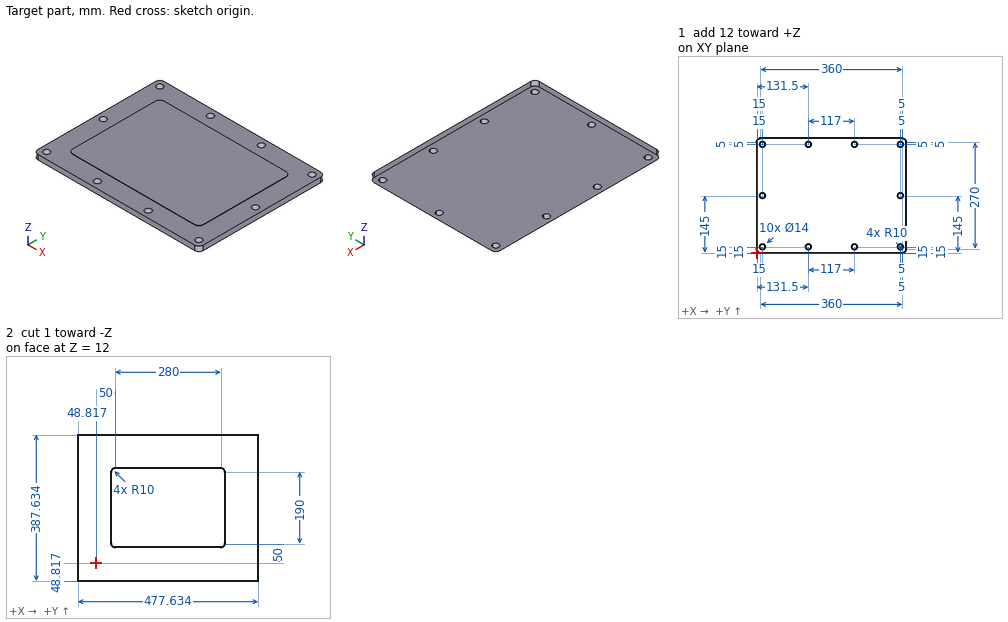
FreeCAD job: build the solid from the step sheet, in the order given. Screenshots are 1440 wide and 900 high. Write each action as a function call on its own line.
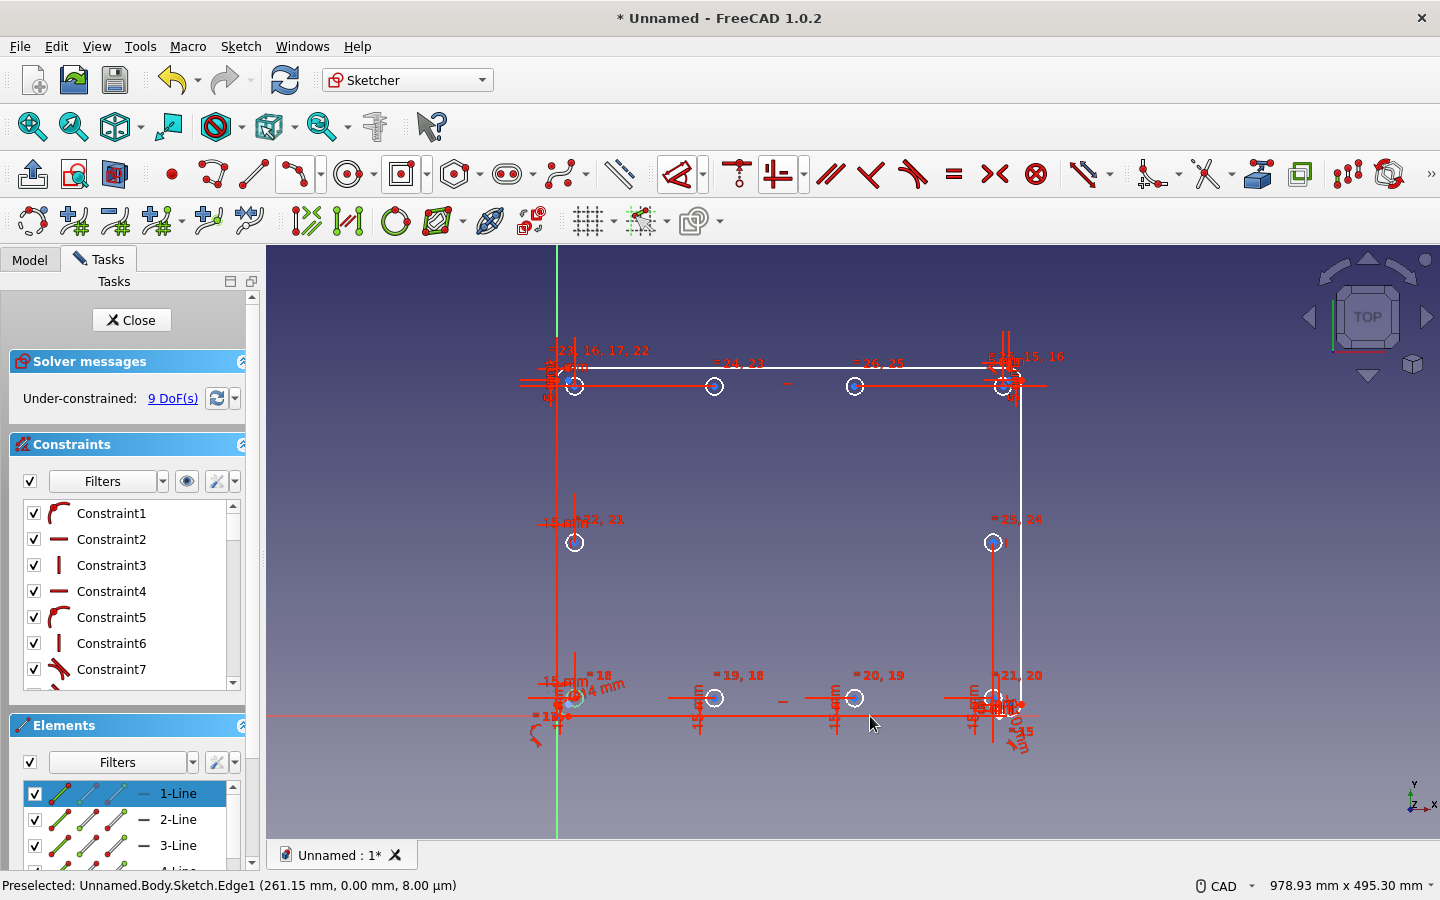
click(702, 174)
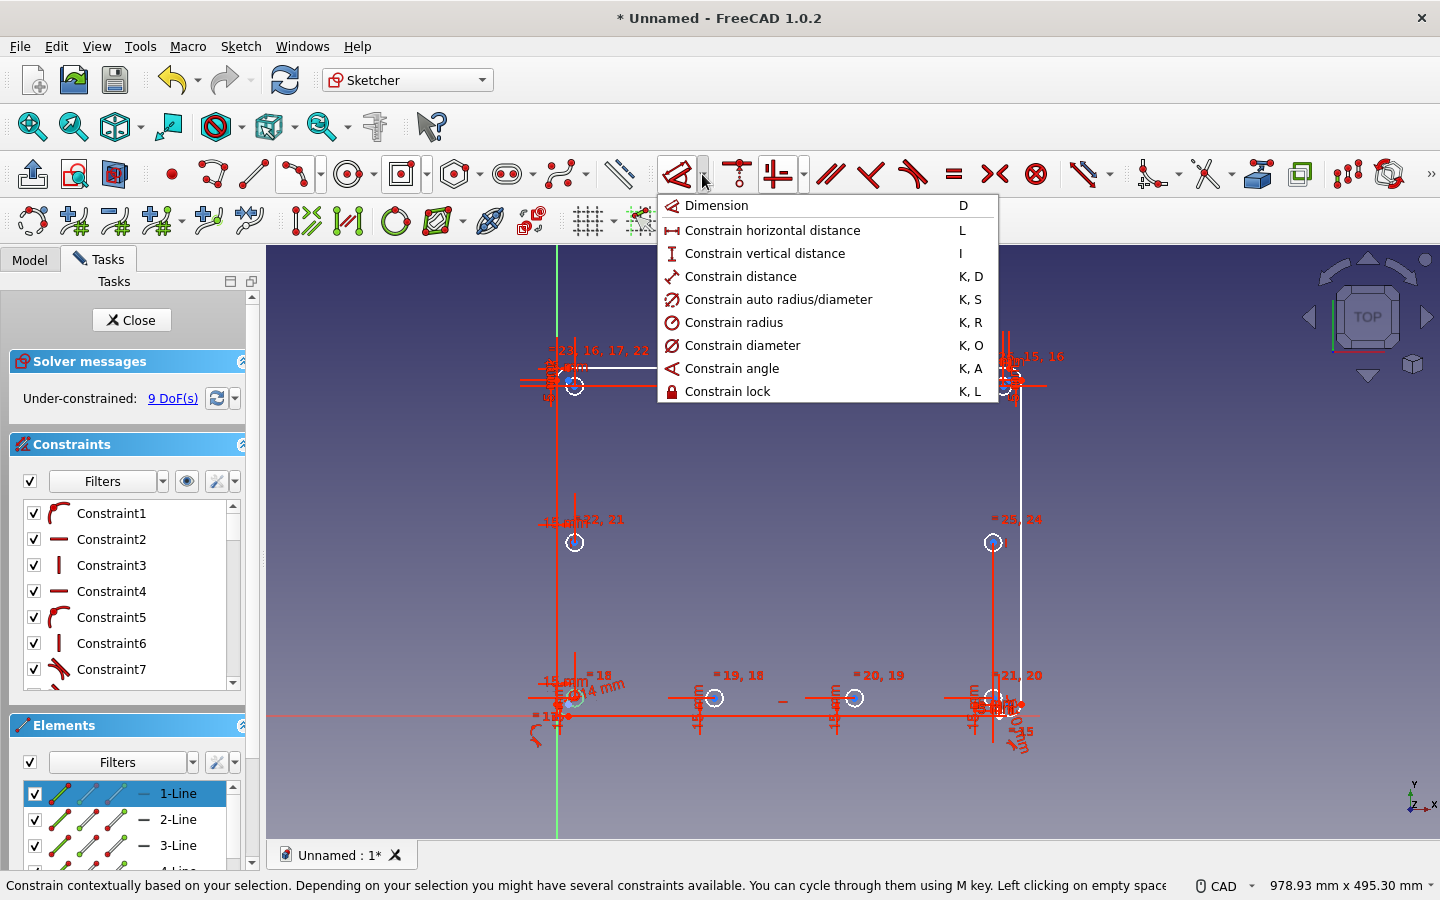
click(828, 230)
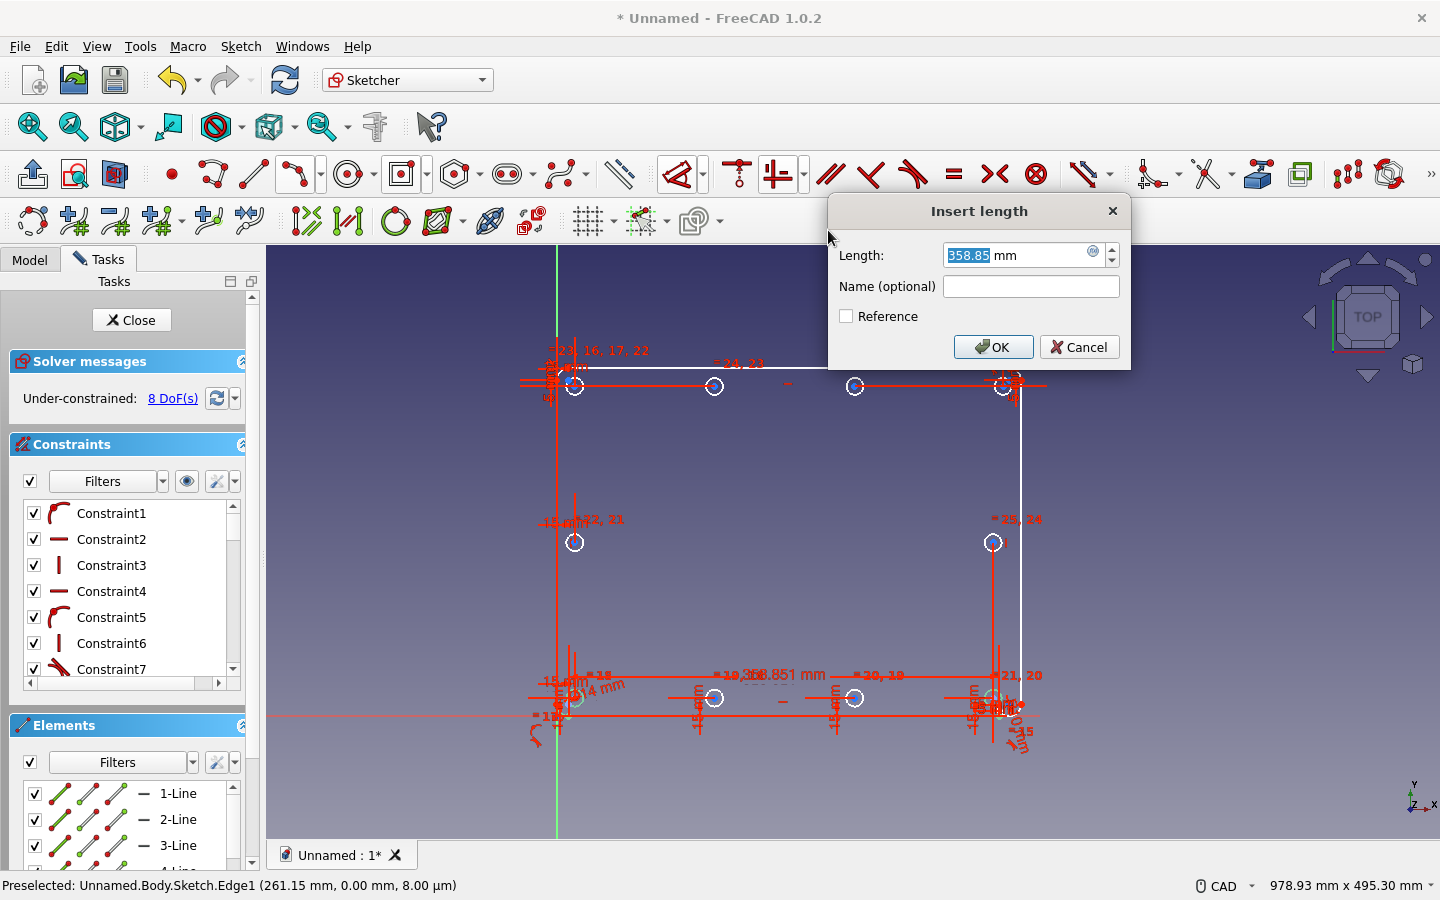
text(360)
key(Return)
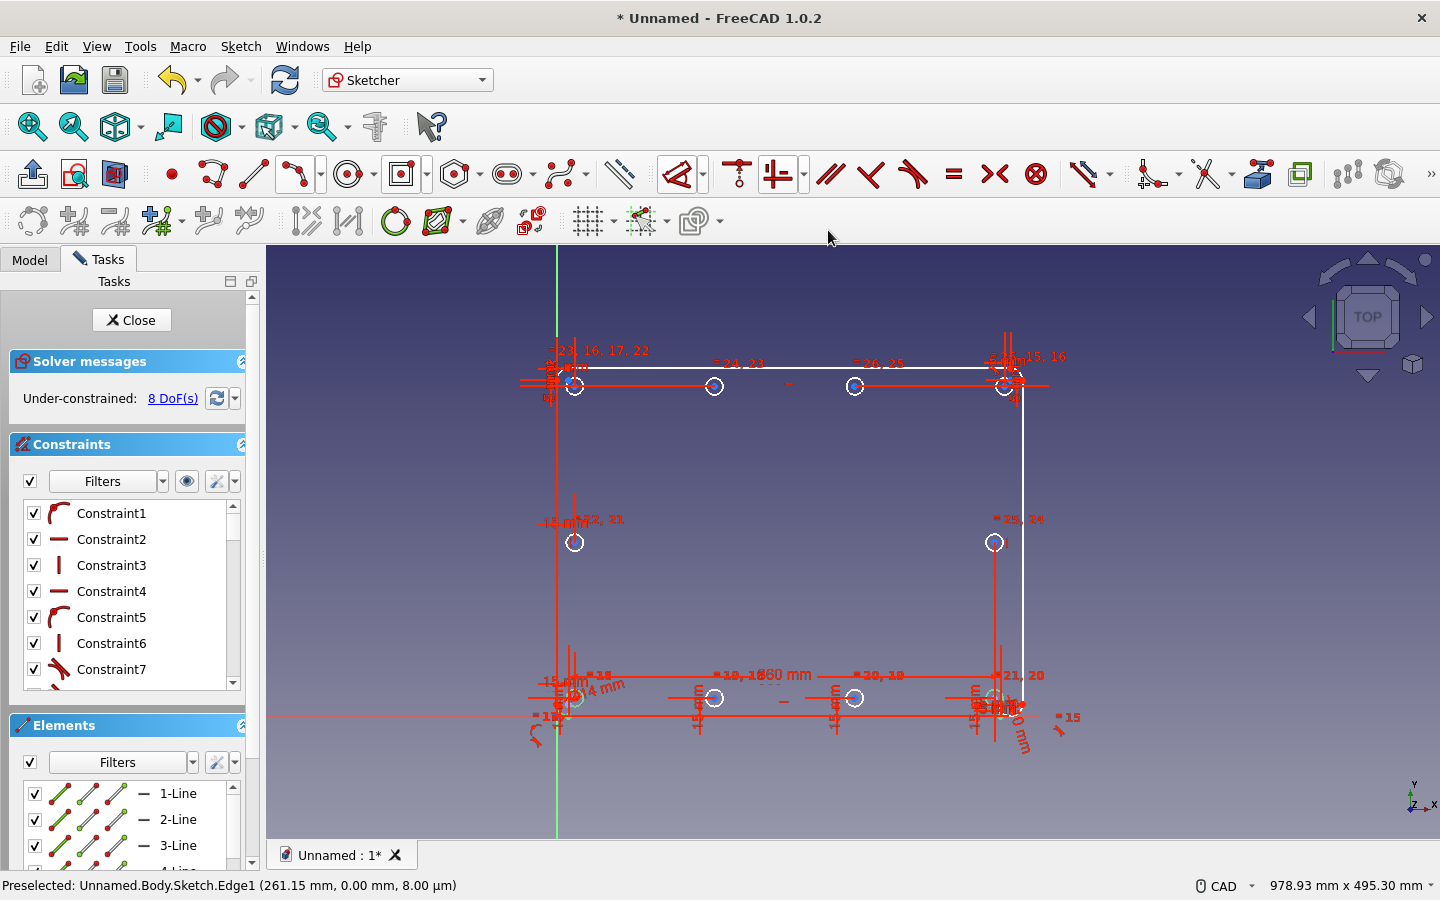
click(1023, 607)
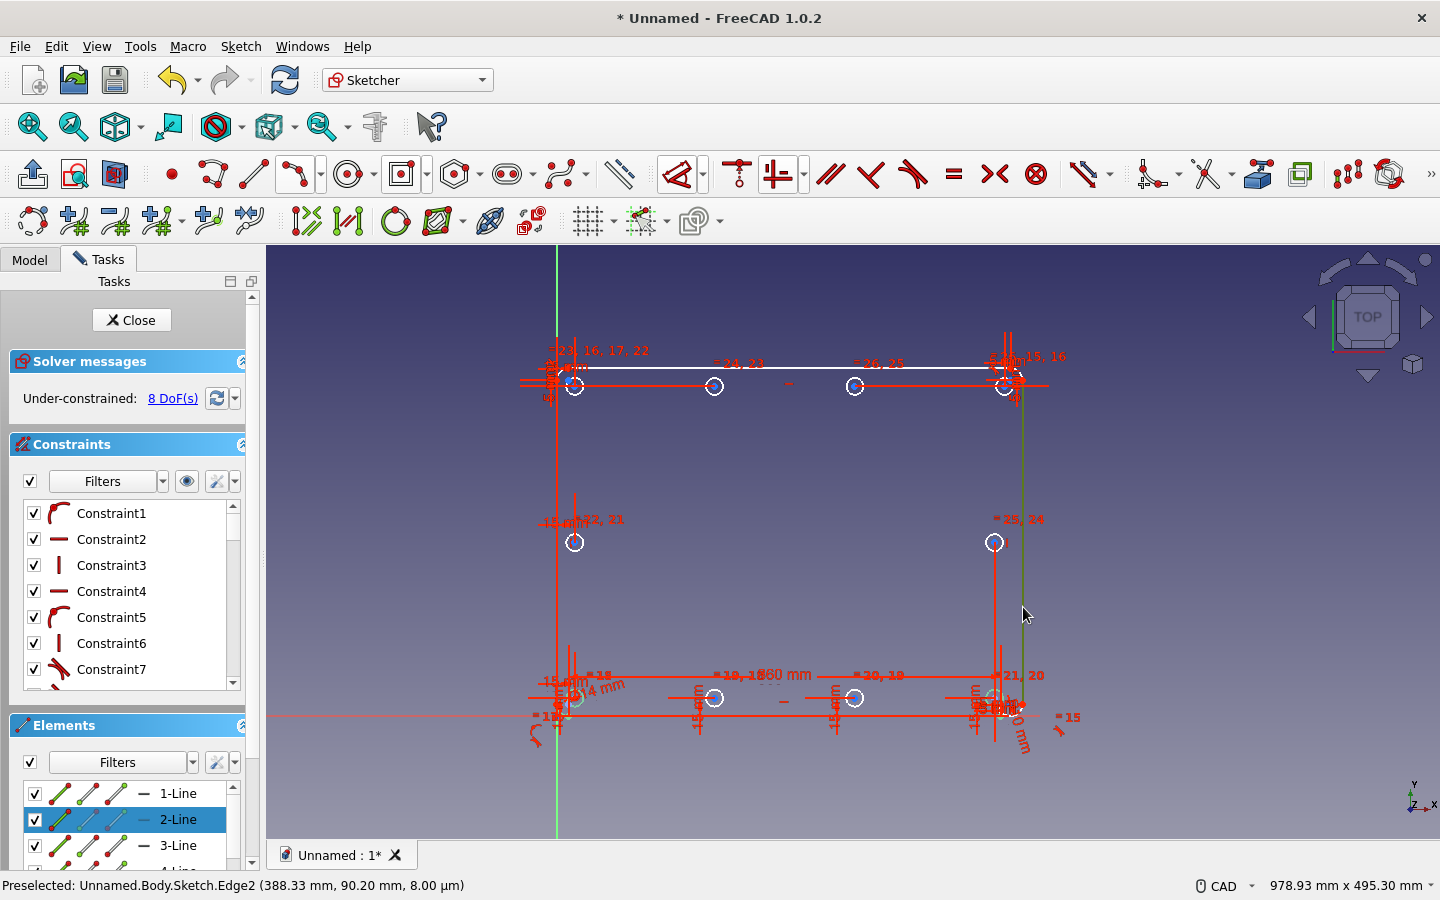
key(i)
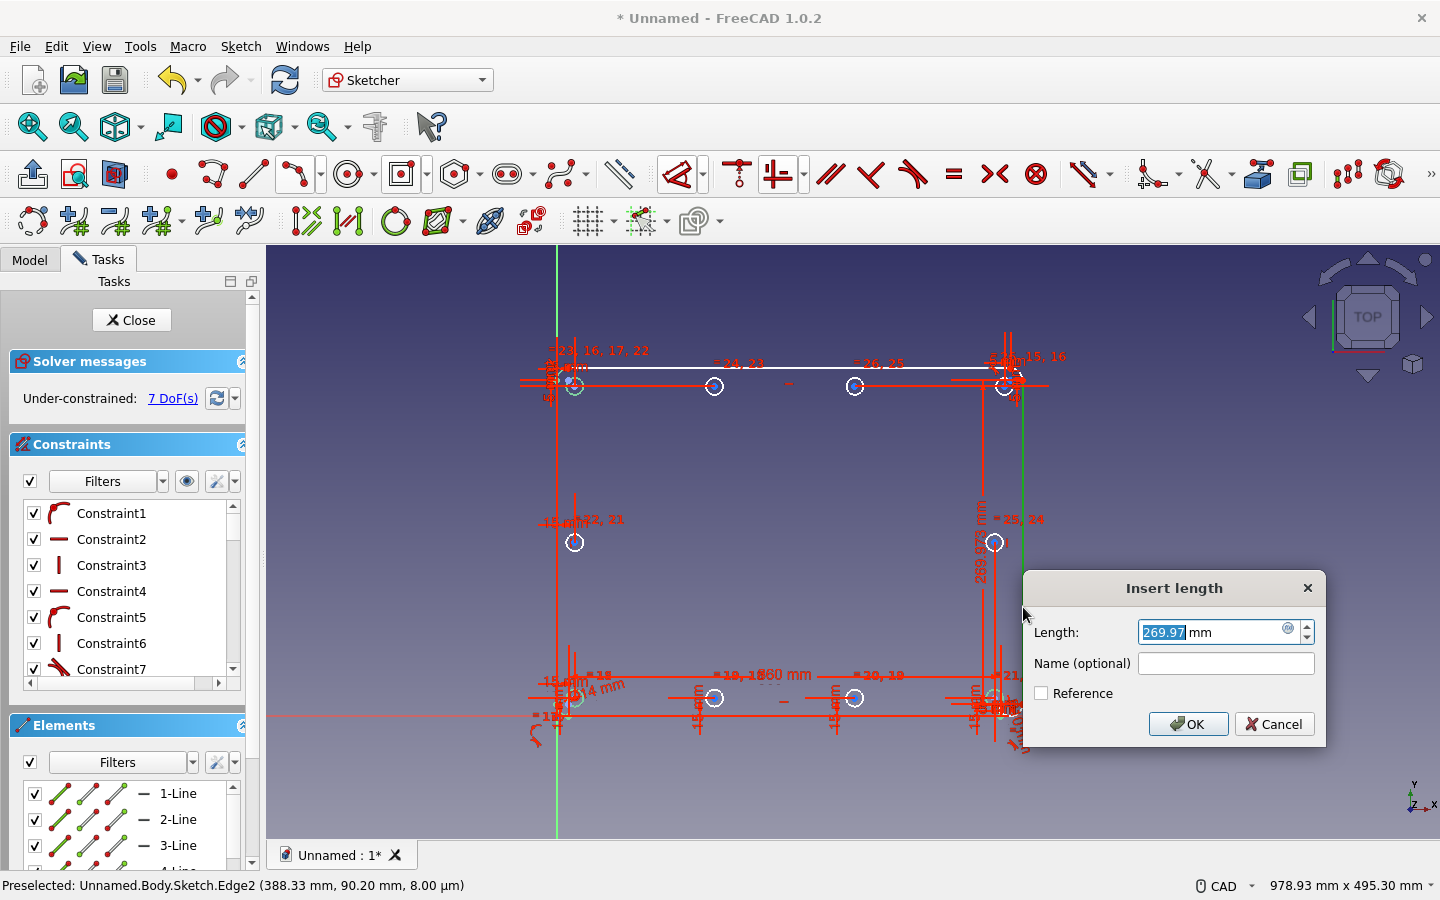
text(270)
key(Return)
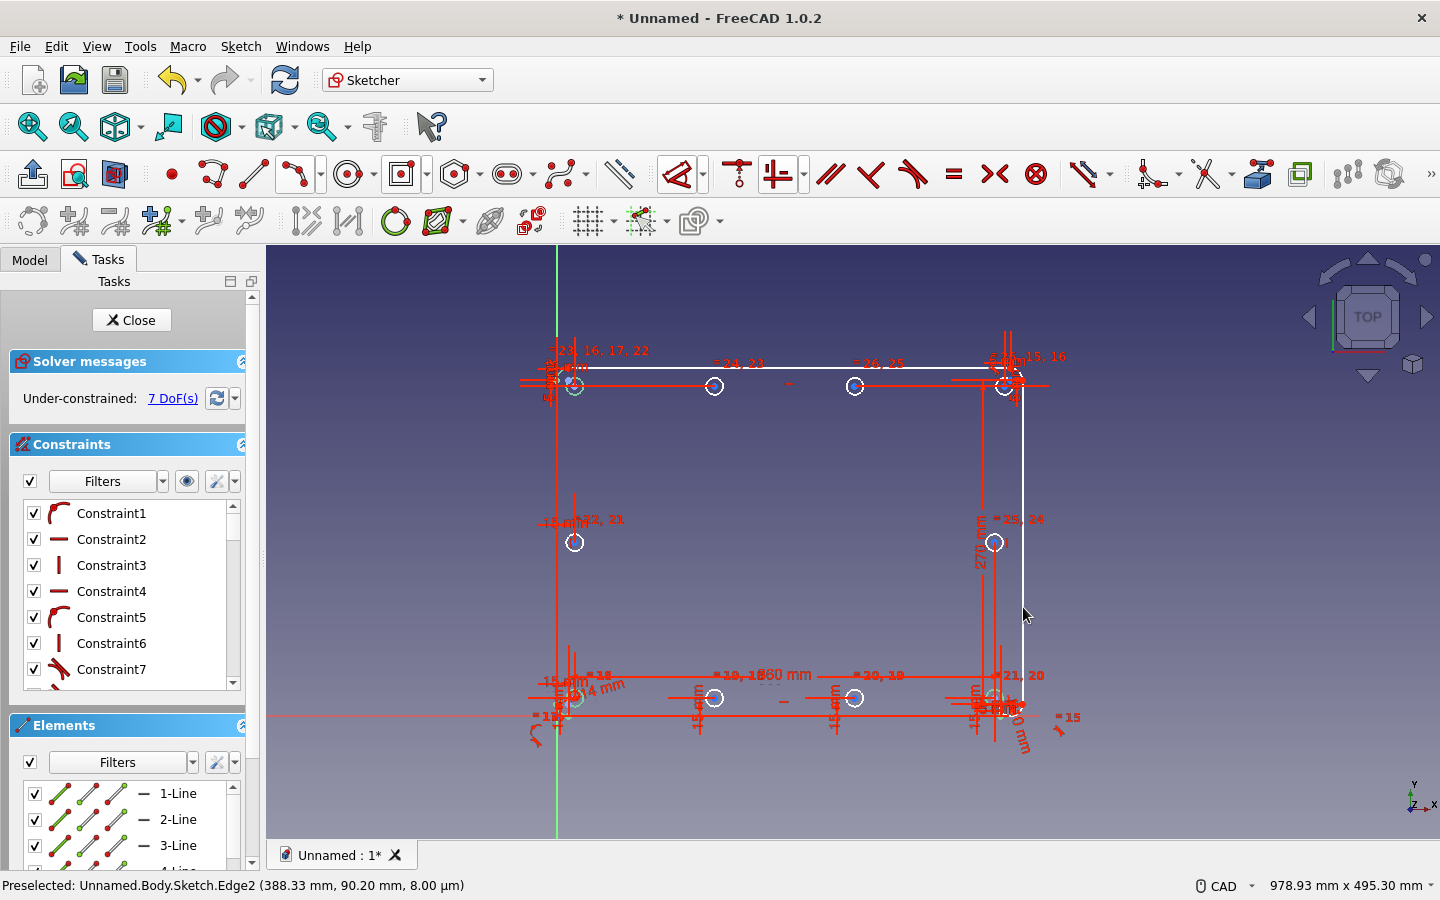
click(701, 368)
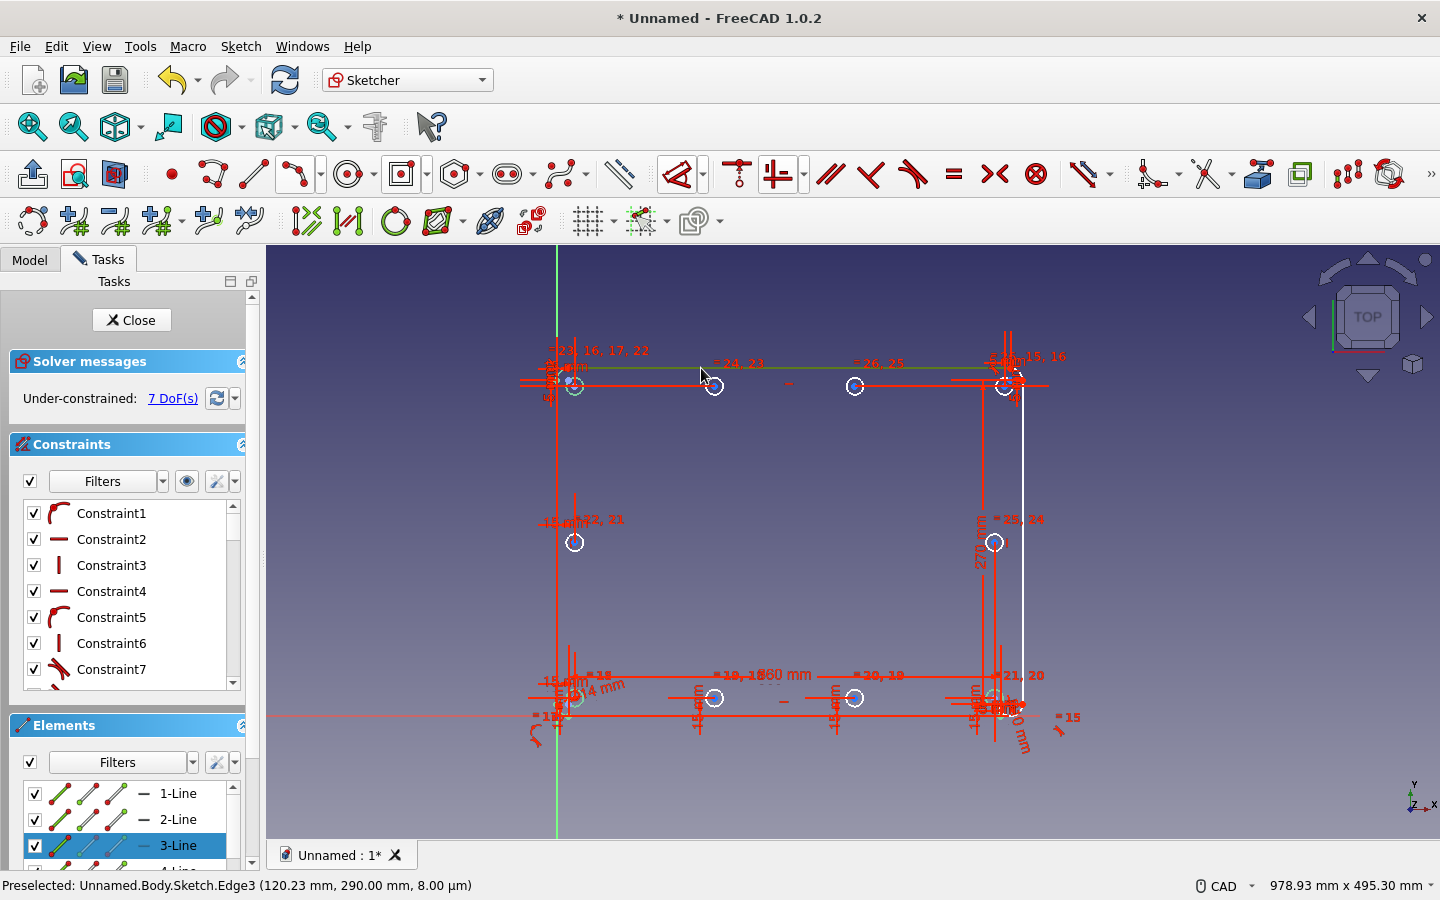
click(702, 174)